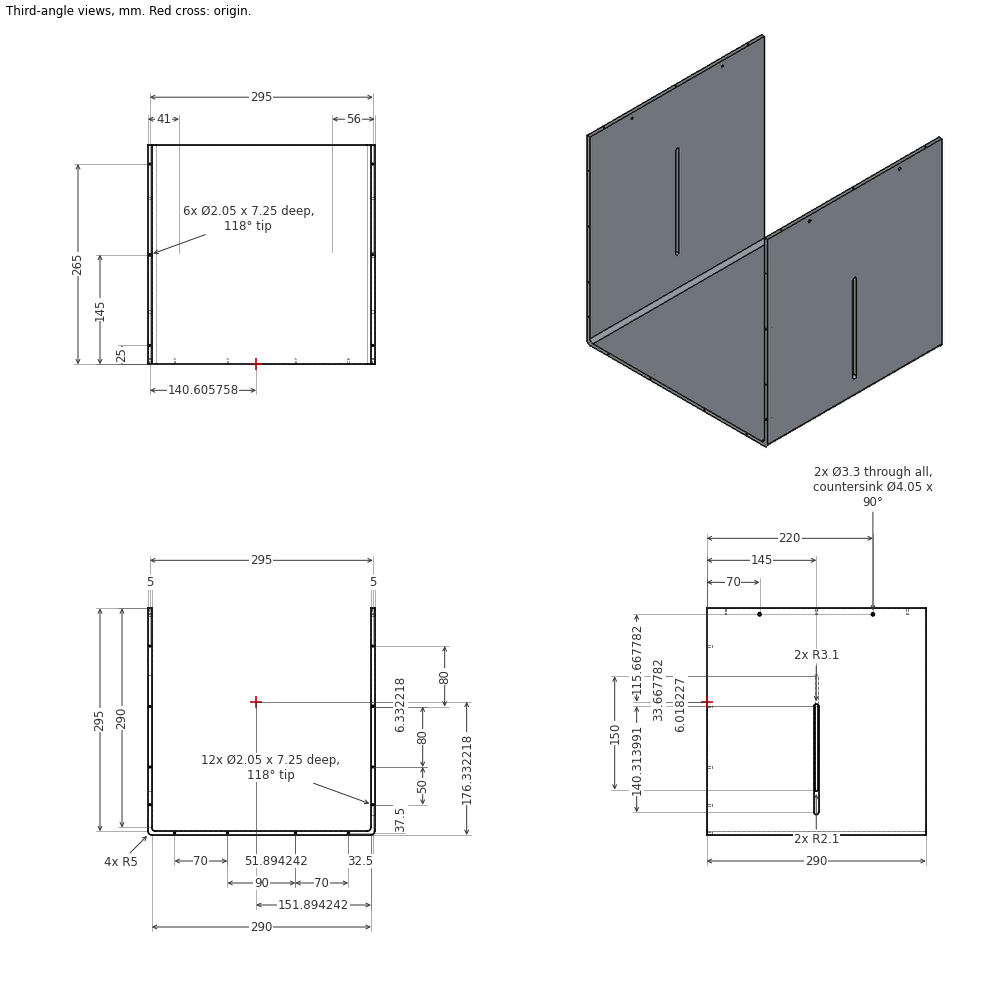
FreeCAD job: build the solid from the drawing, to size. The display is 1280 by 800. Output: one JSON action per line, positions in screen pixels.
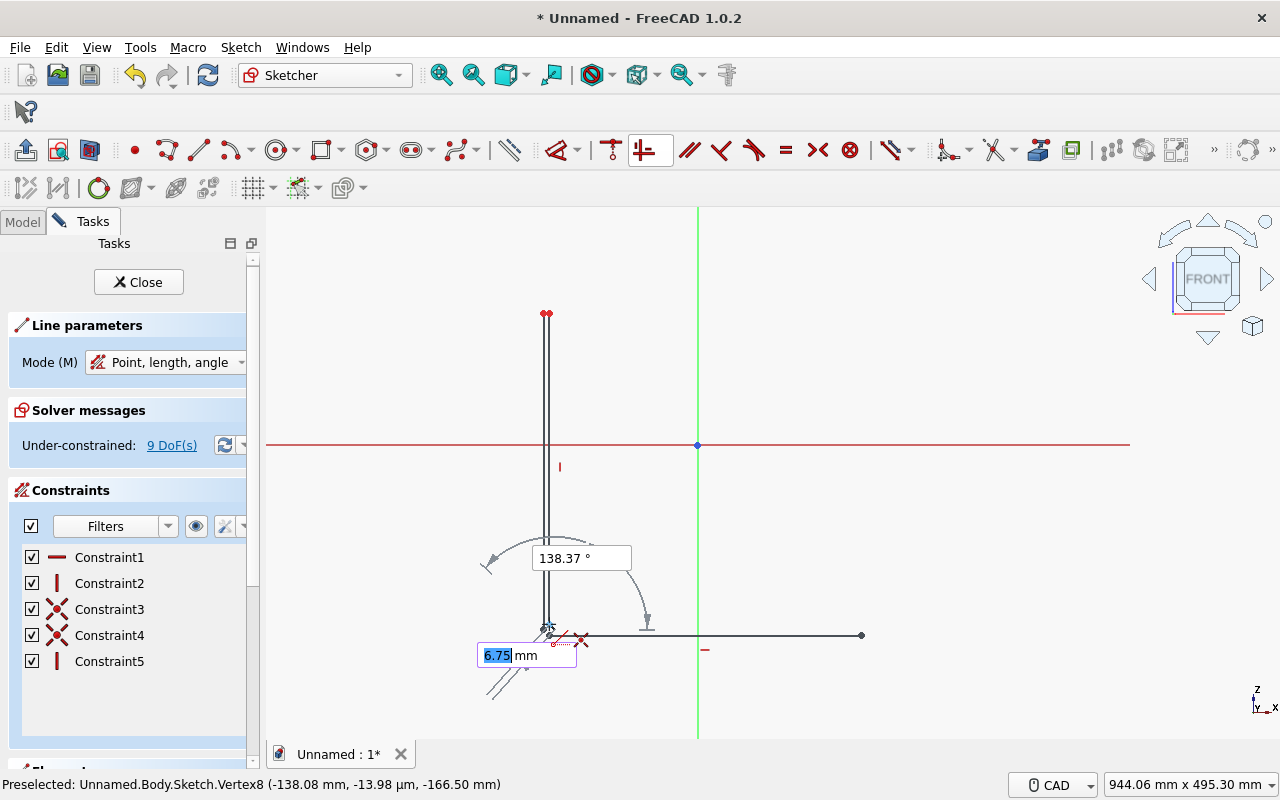
{"action": "scroll", "coordinate": [855, 629], "scroll_direction": "up", "scroll_amount": 6}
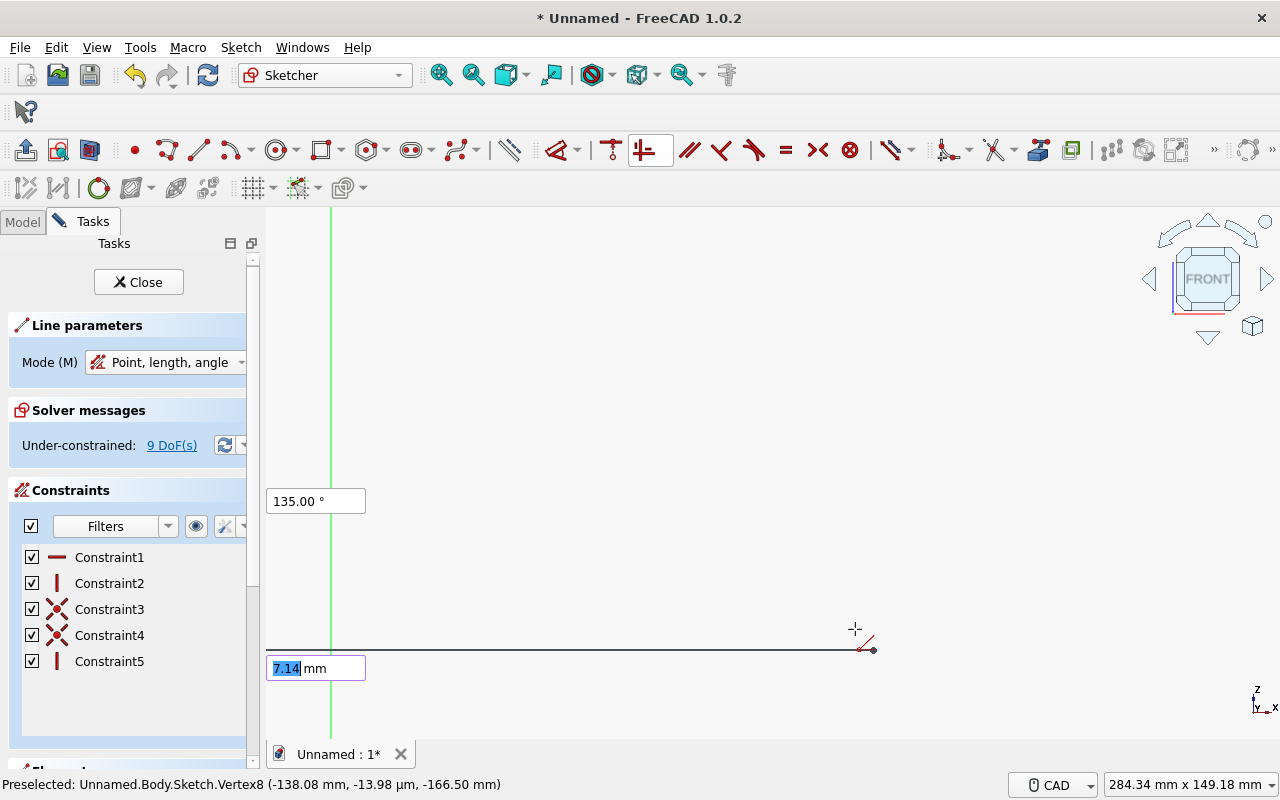
{"action": "left_click", "coordinate": [855, 628]}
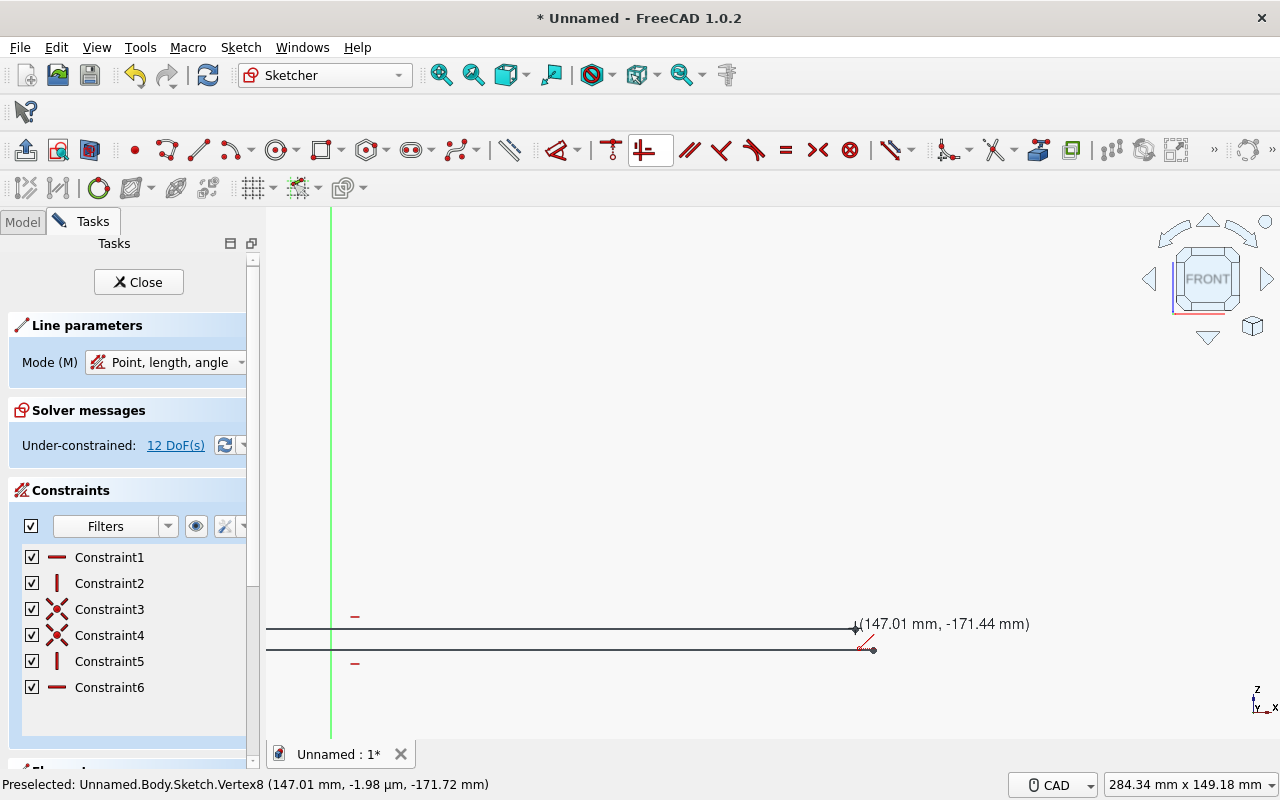
{"action": "left_click", "coordinate": [168, 150]}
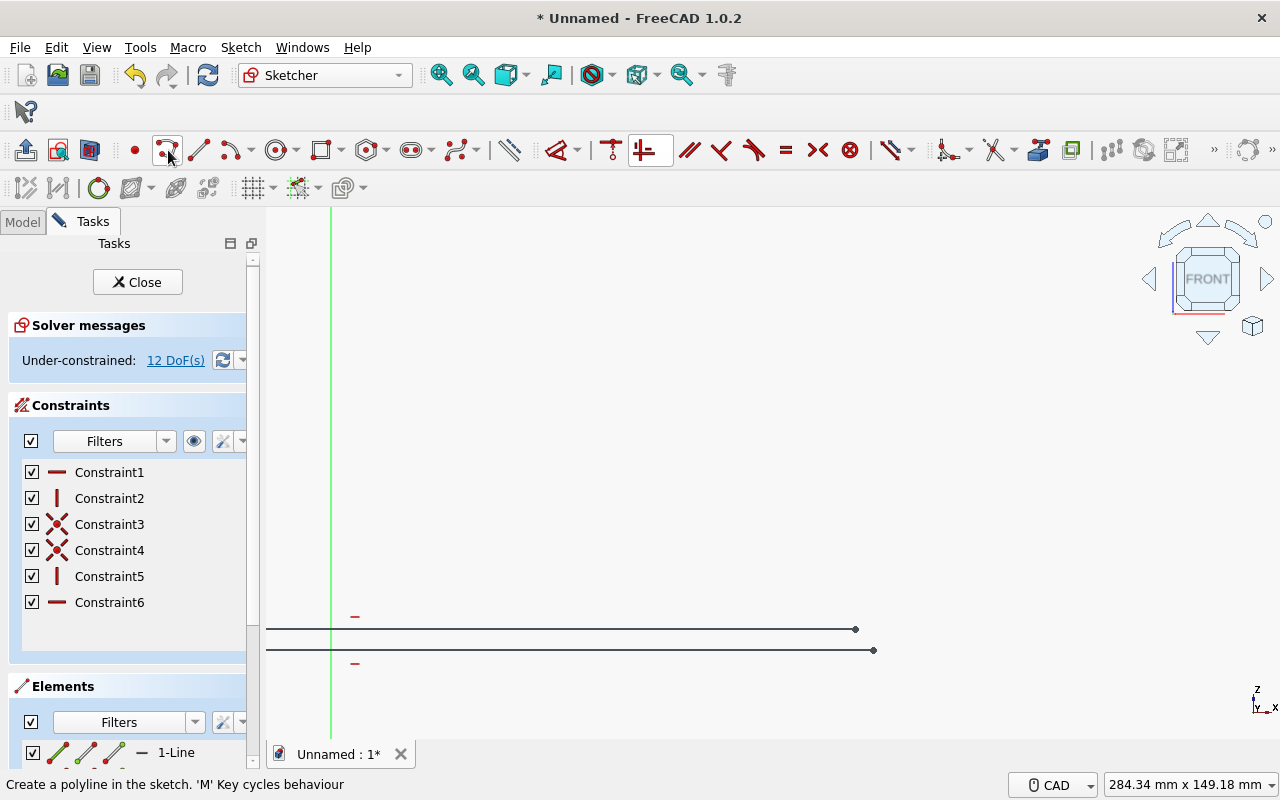
{"action": "left_click", "coordinate": [872, 611]}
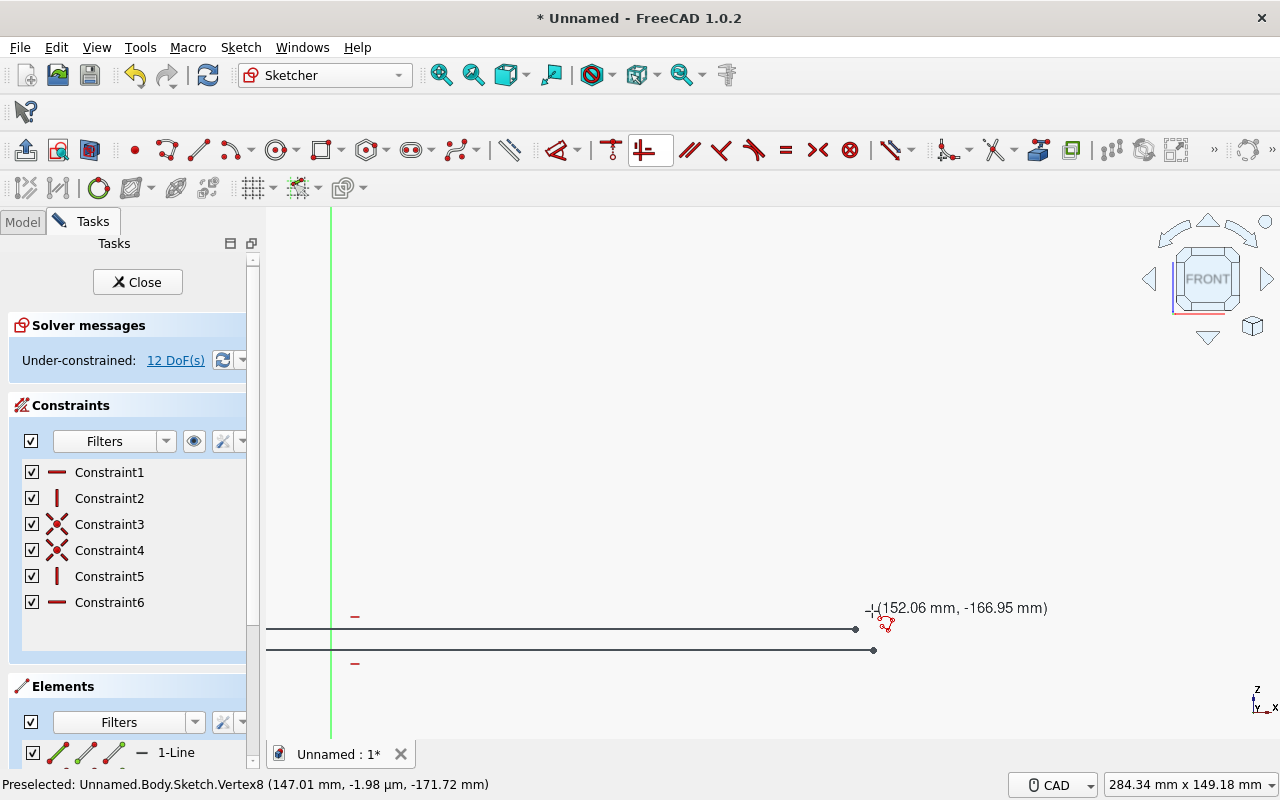
{"action": "scroll", "coordinate": [855, 629], "scroll_direction": "down", "scroll_amount": 6}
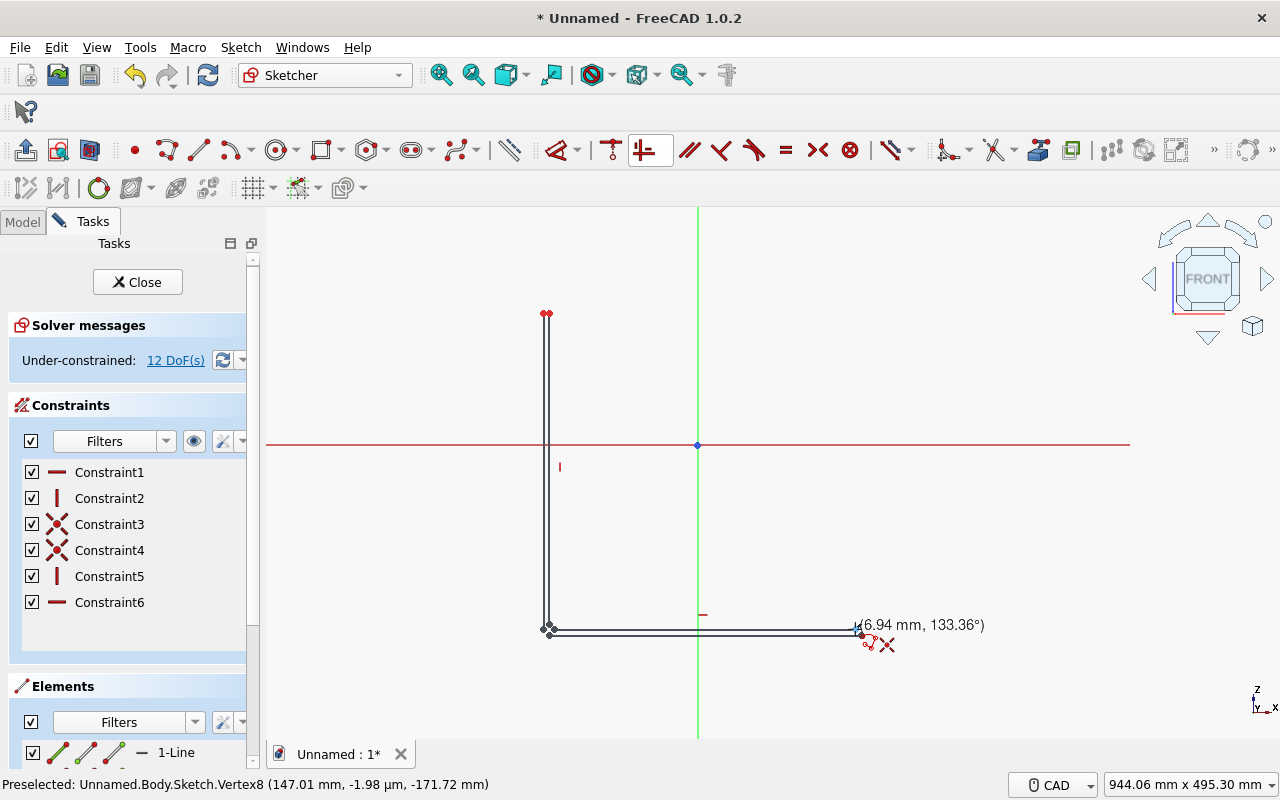
{"action": "left_click", "coordinate": [861, 313]}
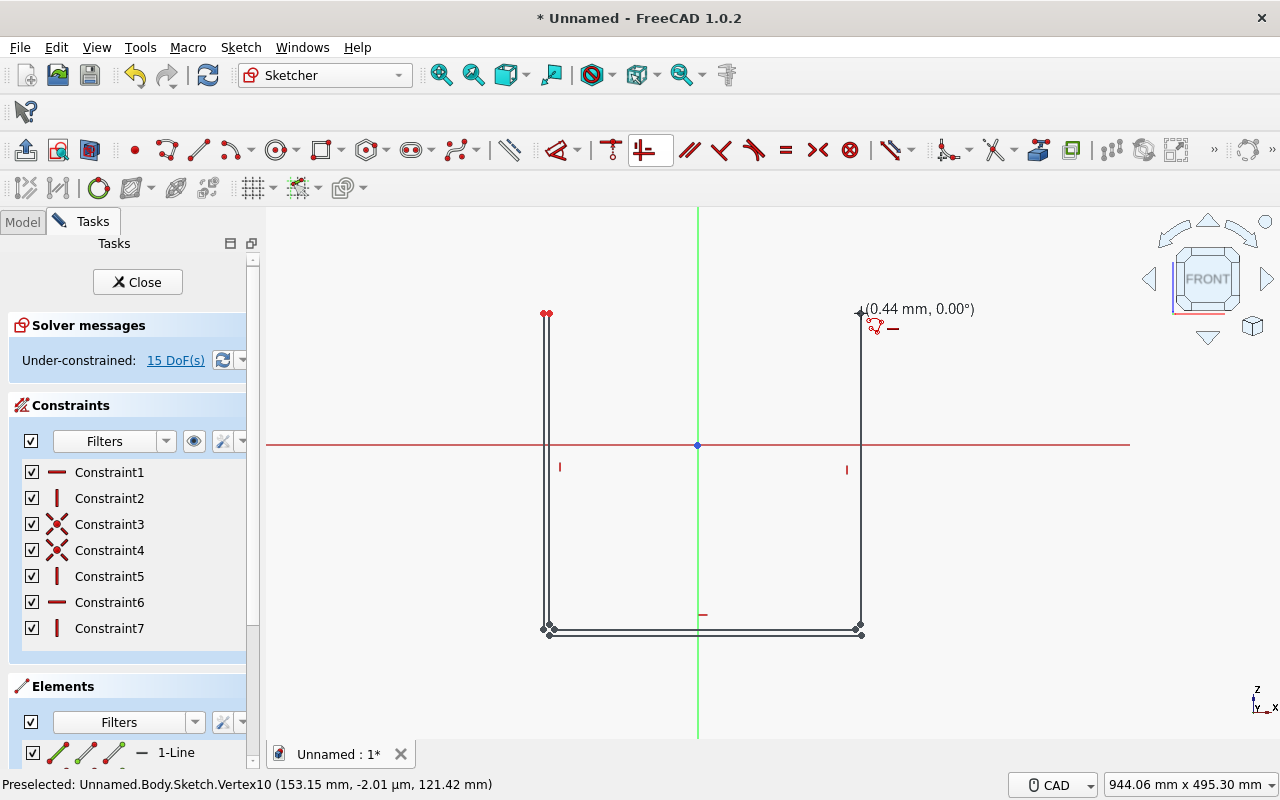
{"action": "scroll", "coordinate": [866, 313], "scroll_direction": "up", "scroll_amount": 6}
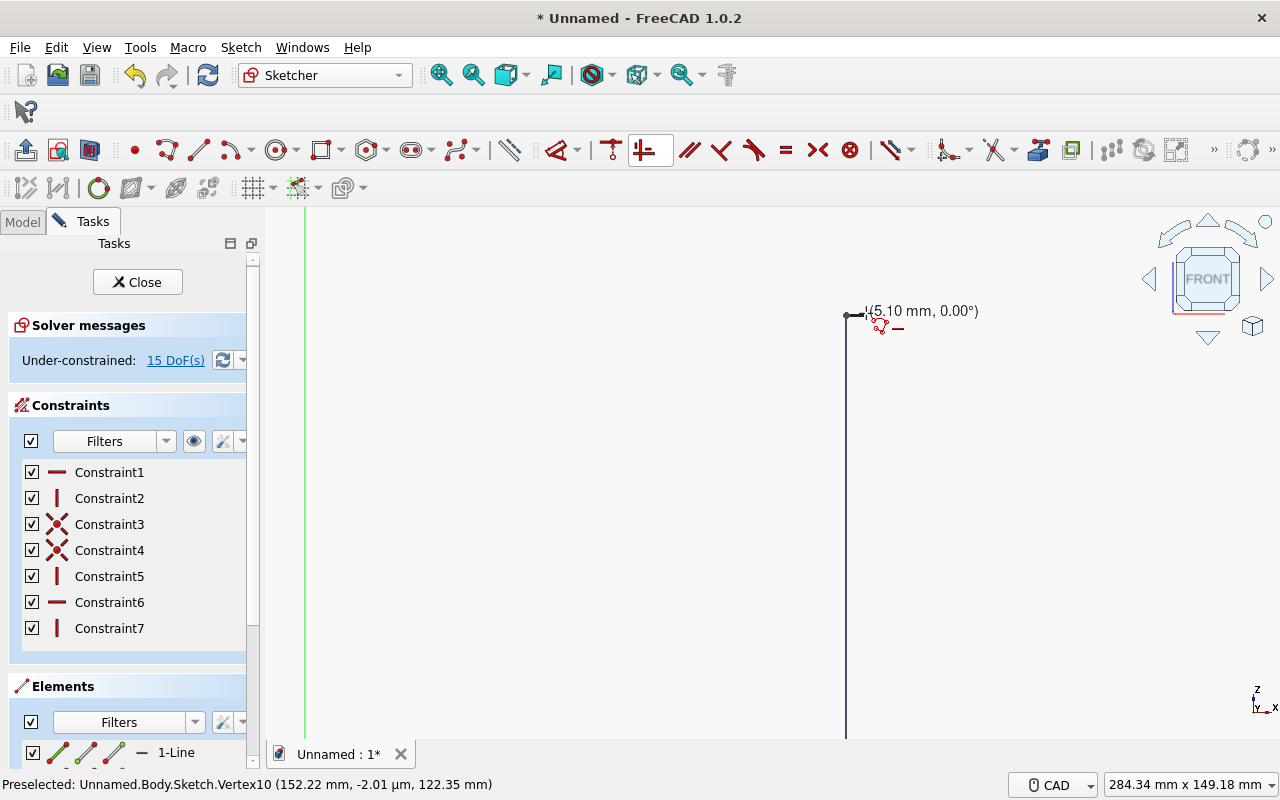
{"action": "left_click", "coordinate": [865, 313]}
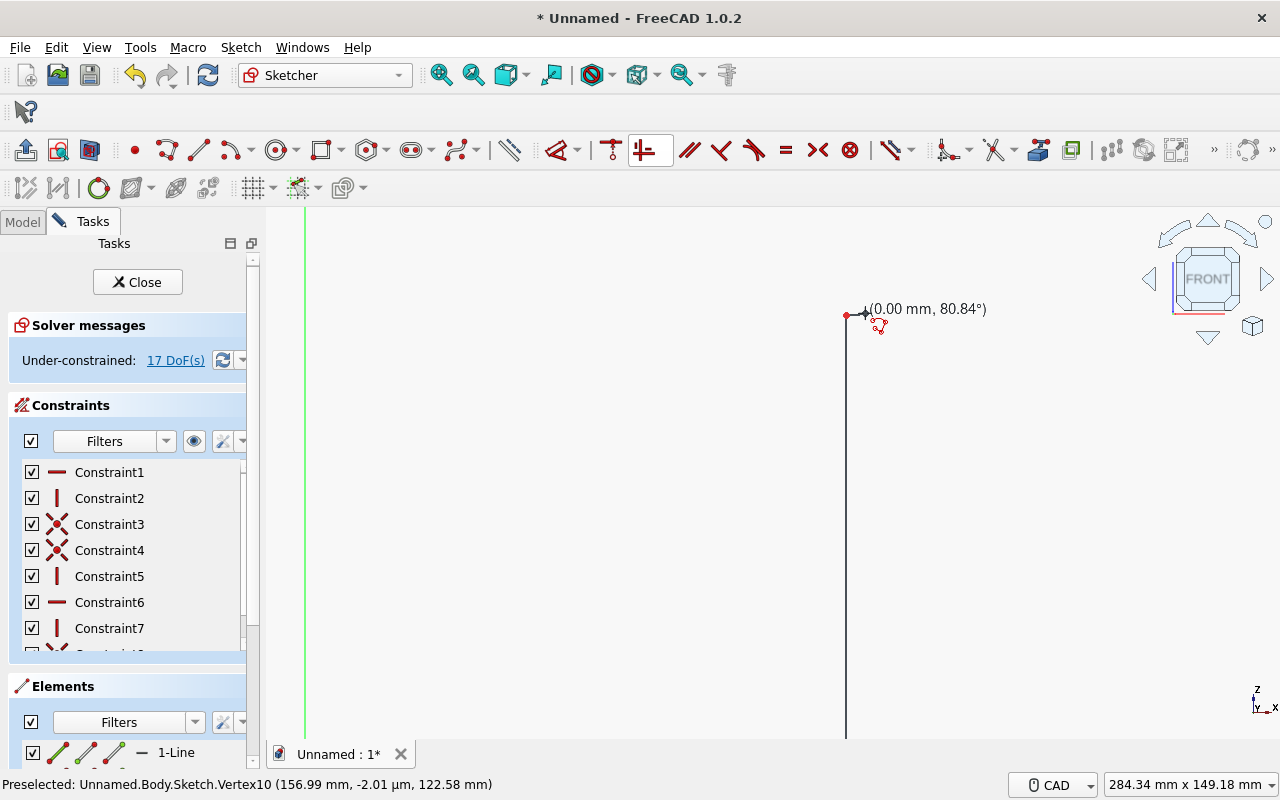
{"action": "scroll", "coordinate": [866, 312], "scroll_direction": "down", "scroll_amount": 6}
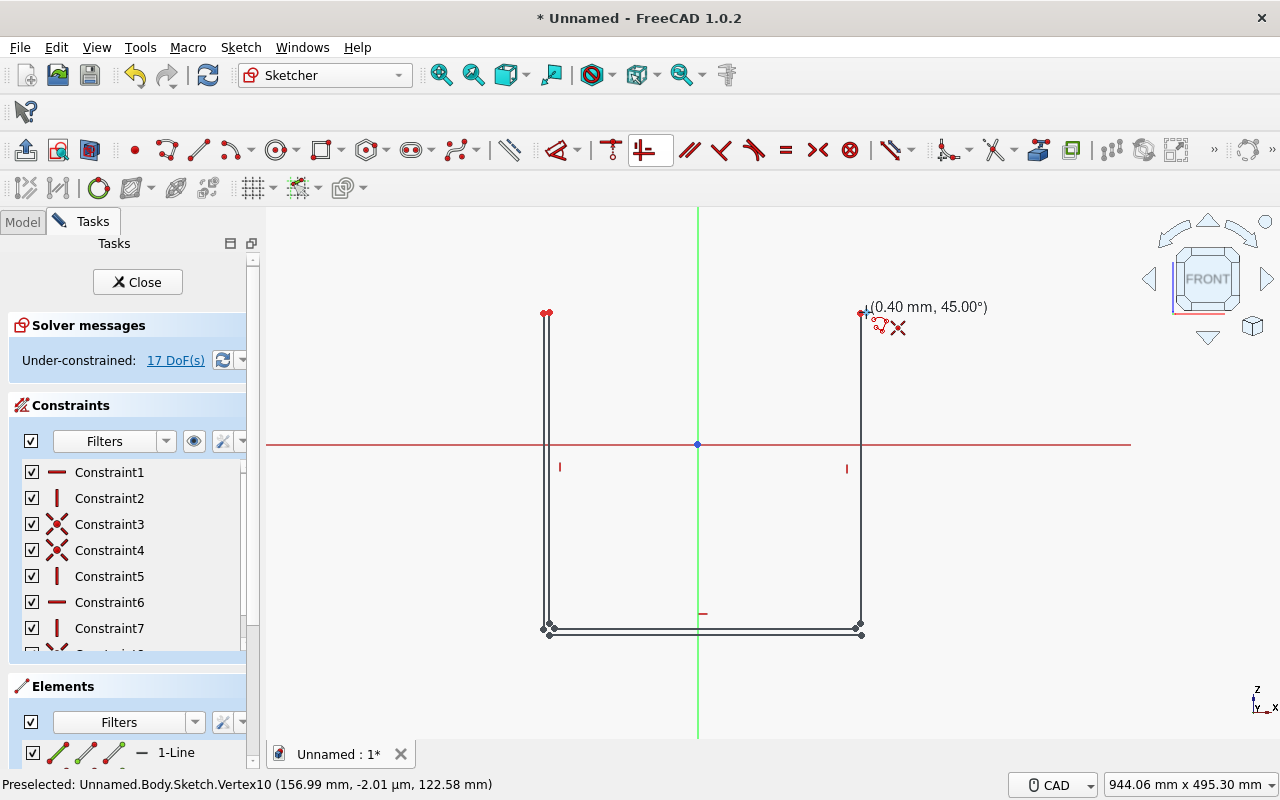
{"action": "scroll", "coordinate": [866, 629], "scroll_direction": "up", "scroll_amount": 4}